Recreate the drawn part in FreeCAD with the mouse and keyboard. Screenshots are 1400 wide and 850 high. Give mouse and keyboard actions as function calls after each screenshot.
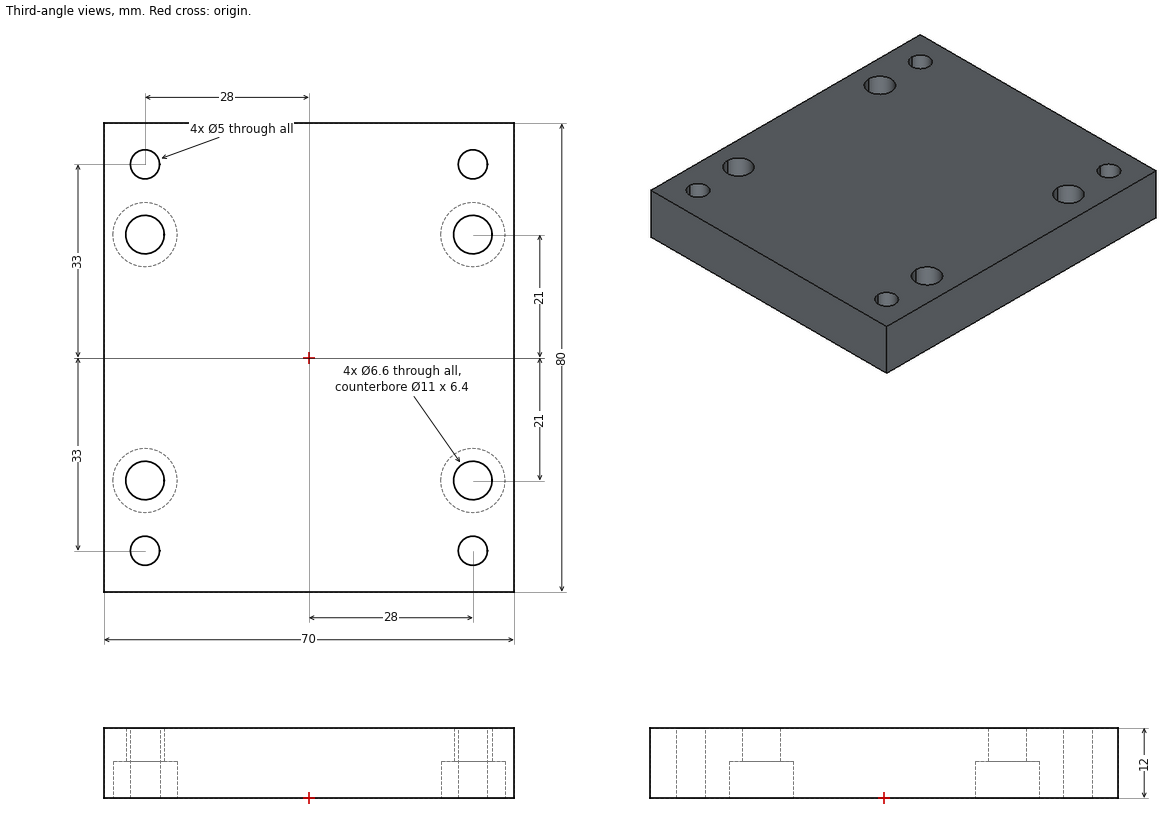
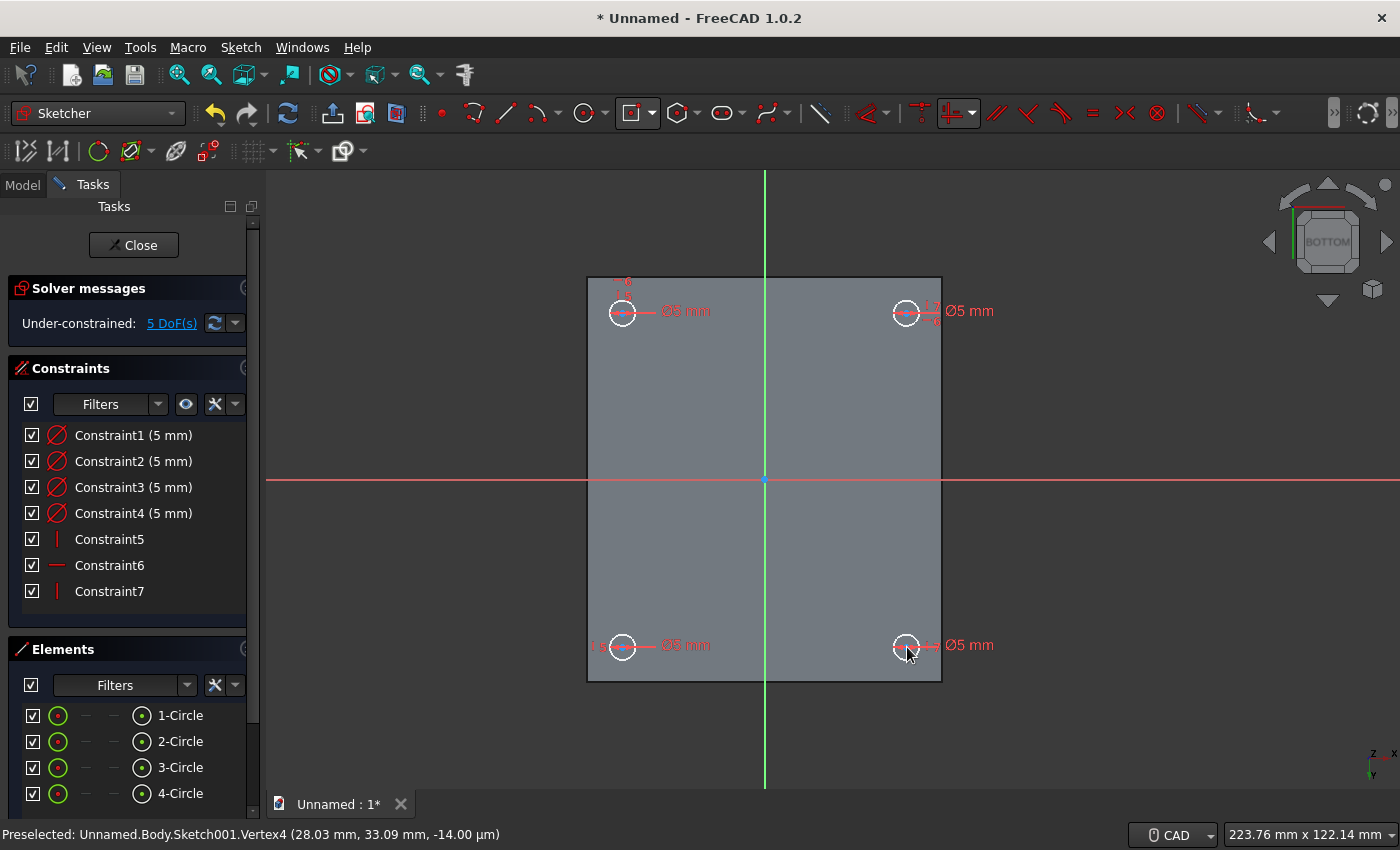
click(623, 647)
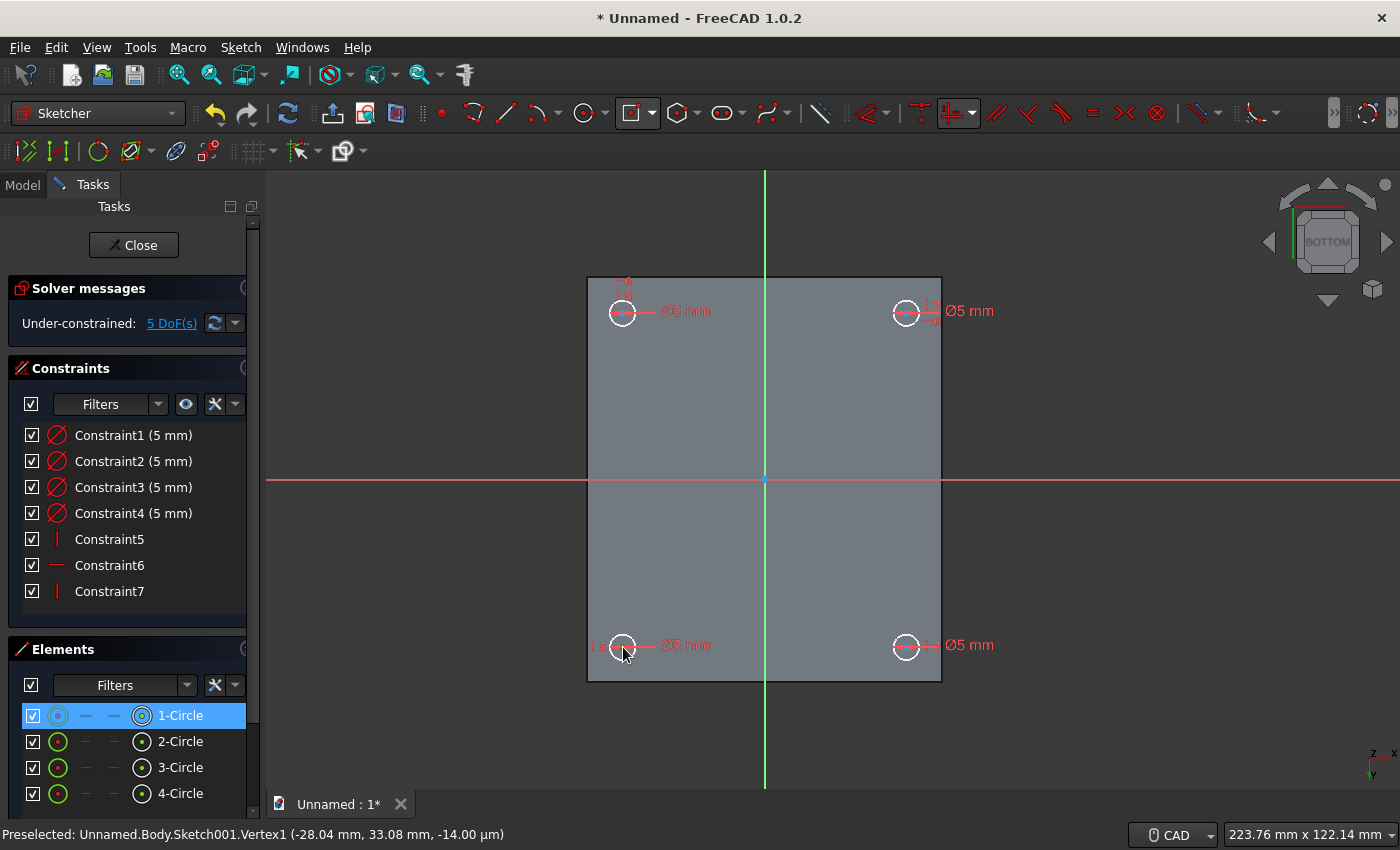
click(906, 647)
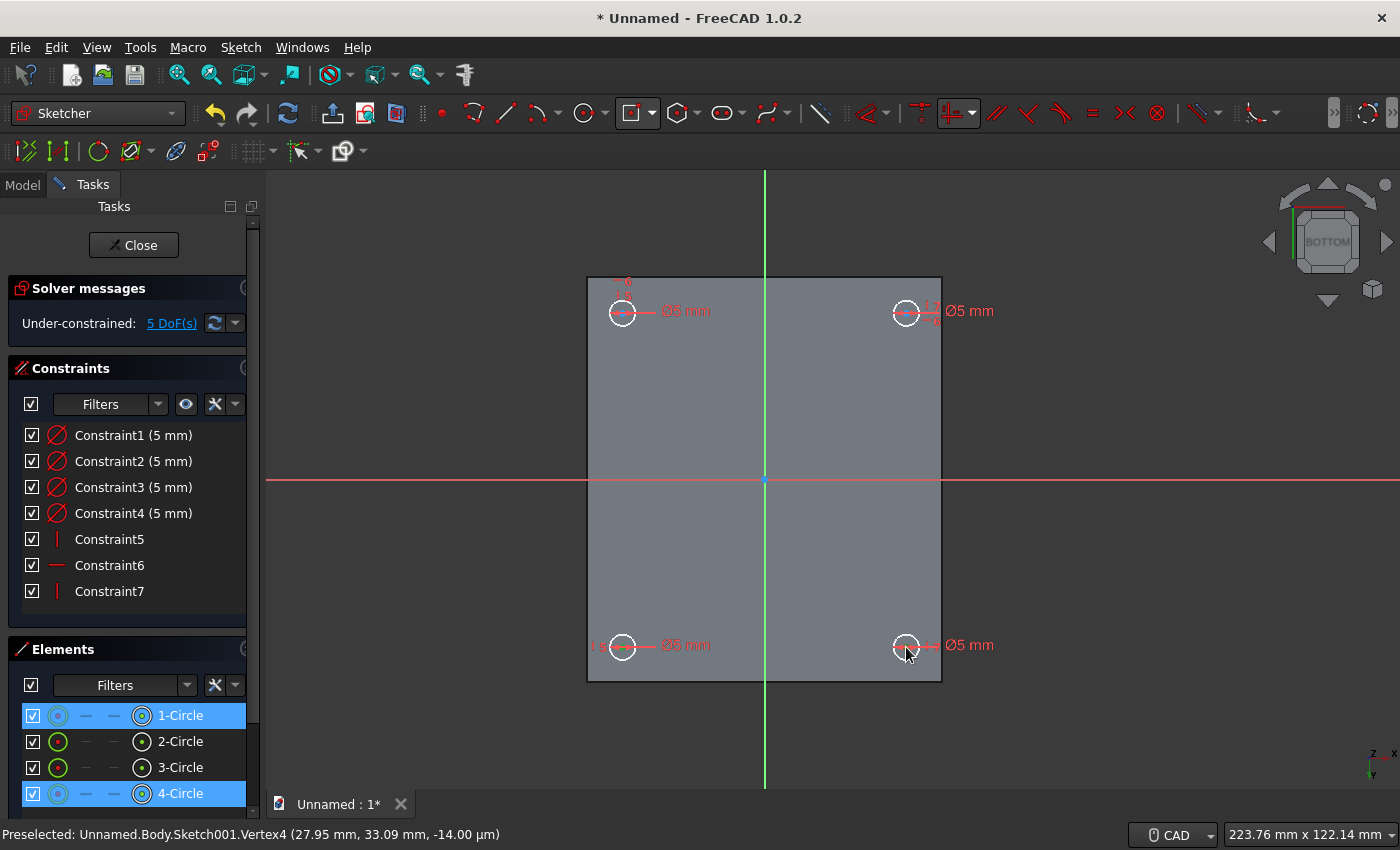
click(974, 114)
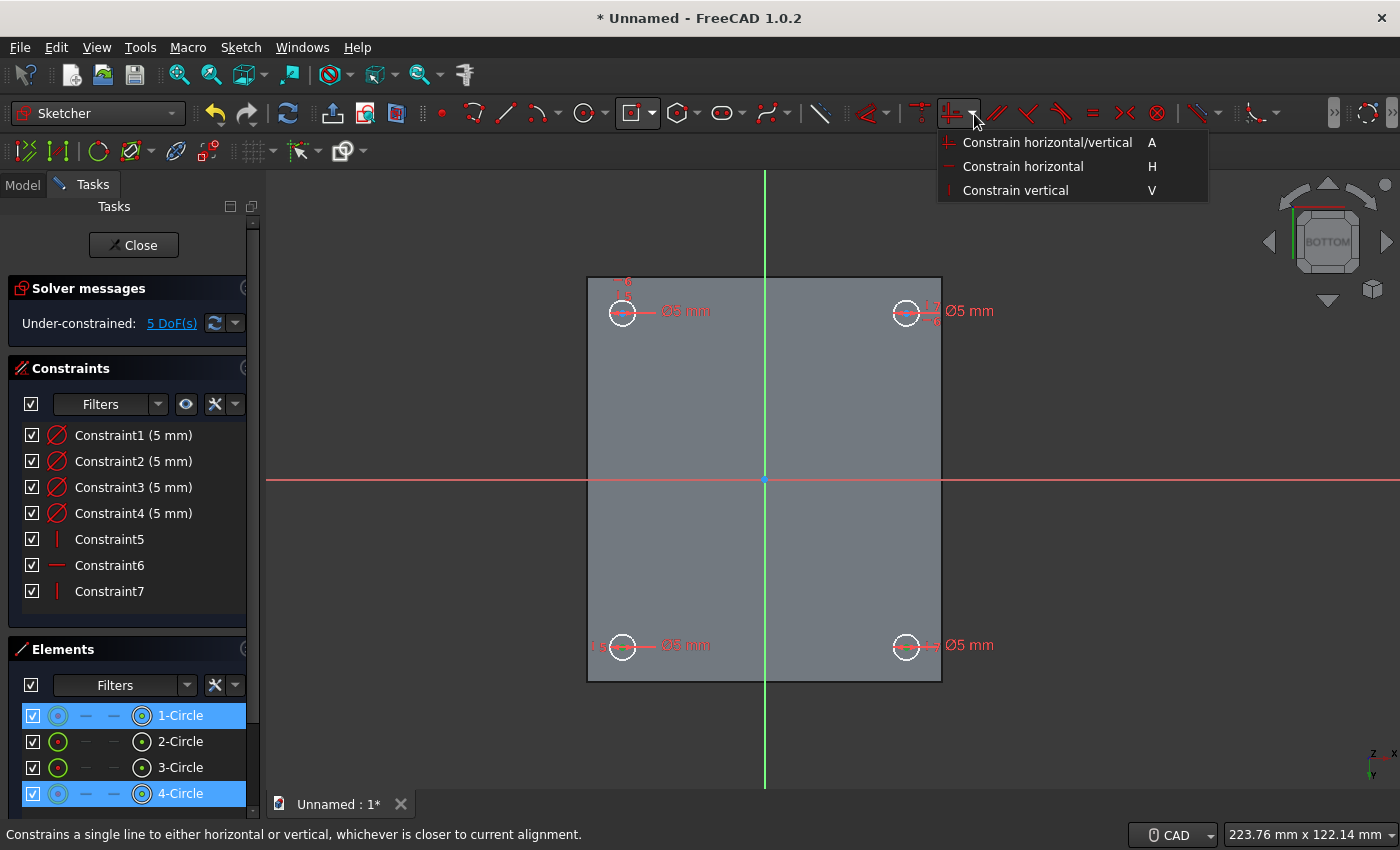
click(1073, 166)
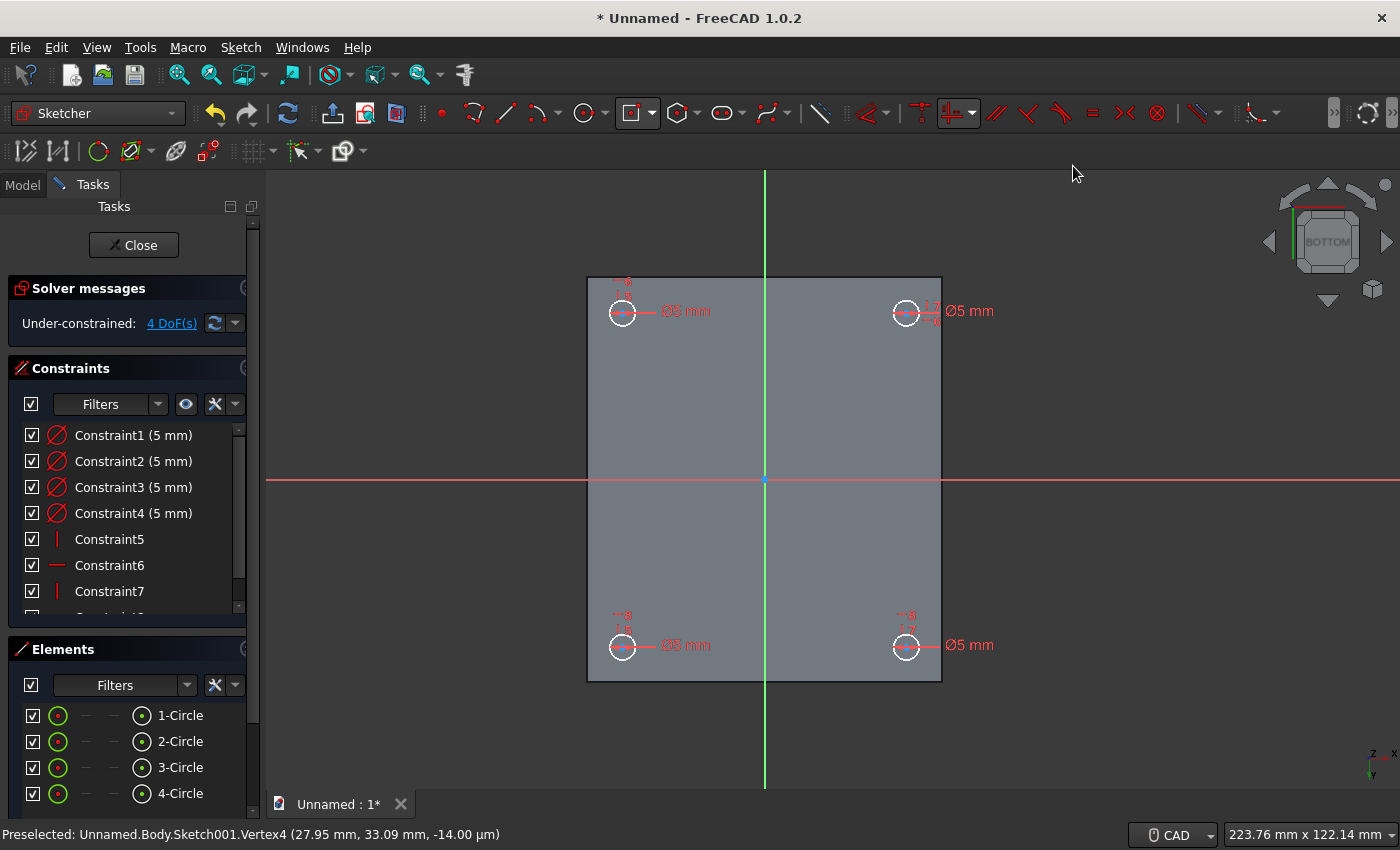
click(623, 647)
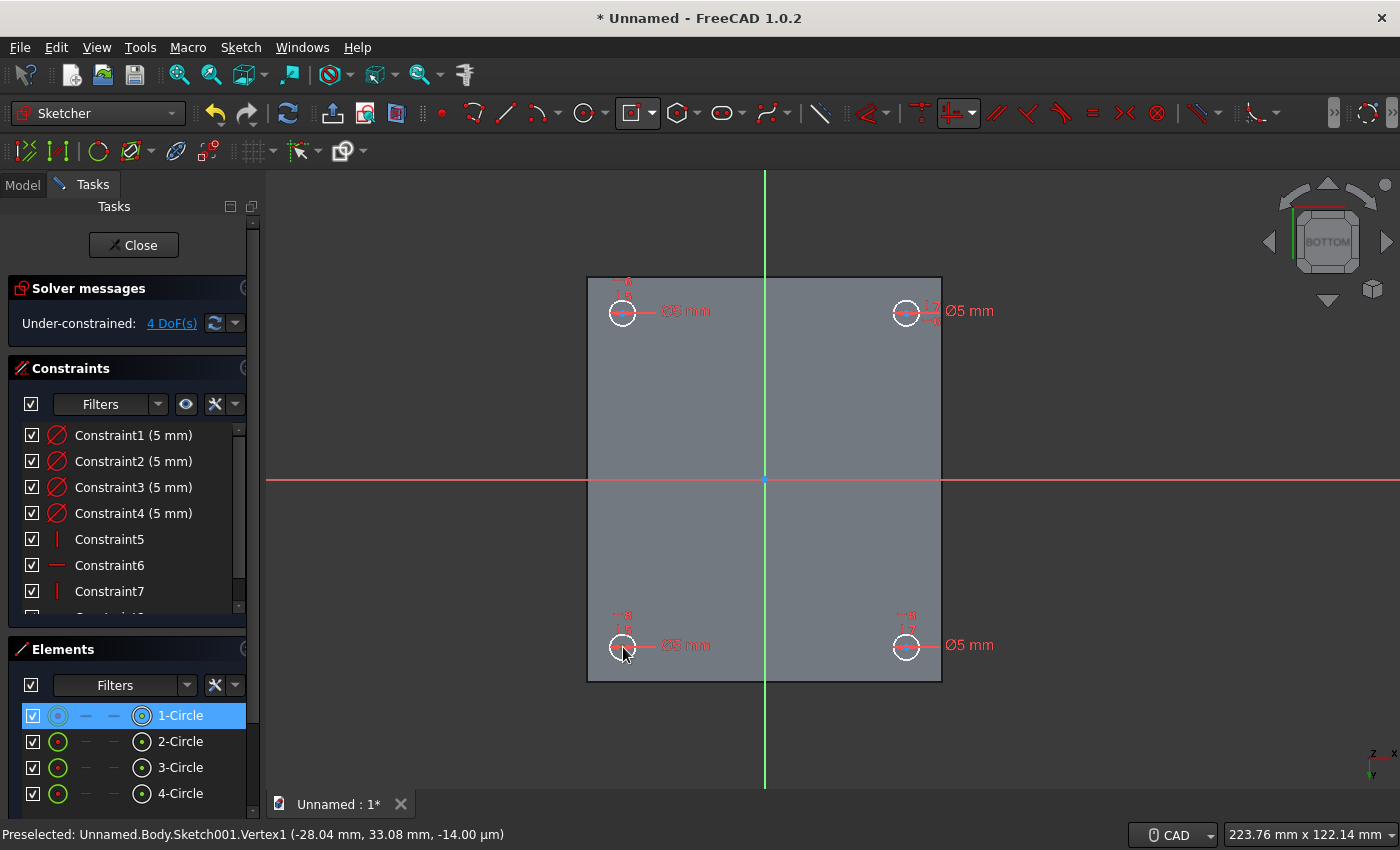
click(888, 114)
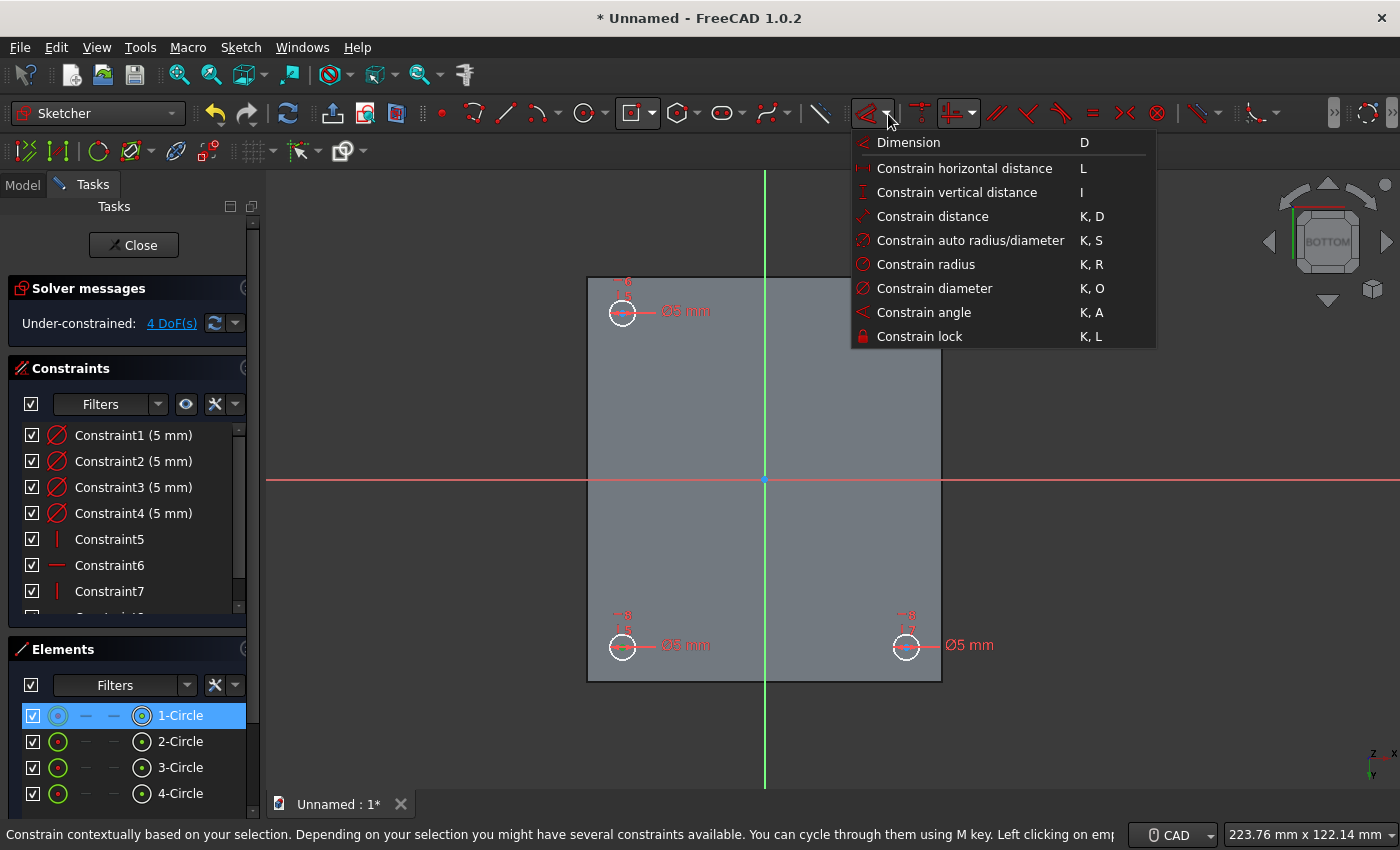
click(1004, 168)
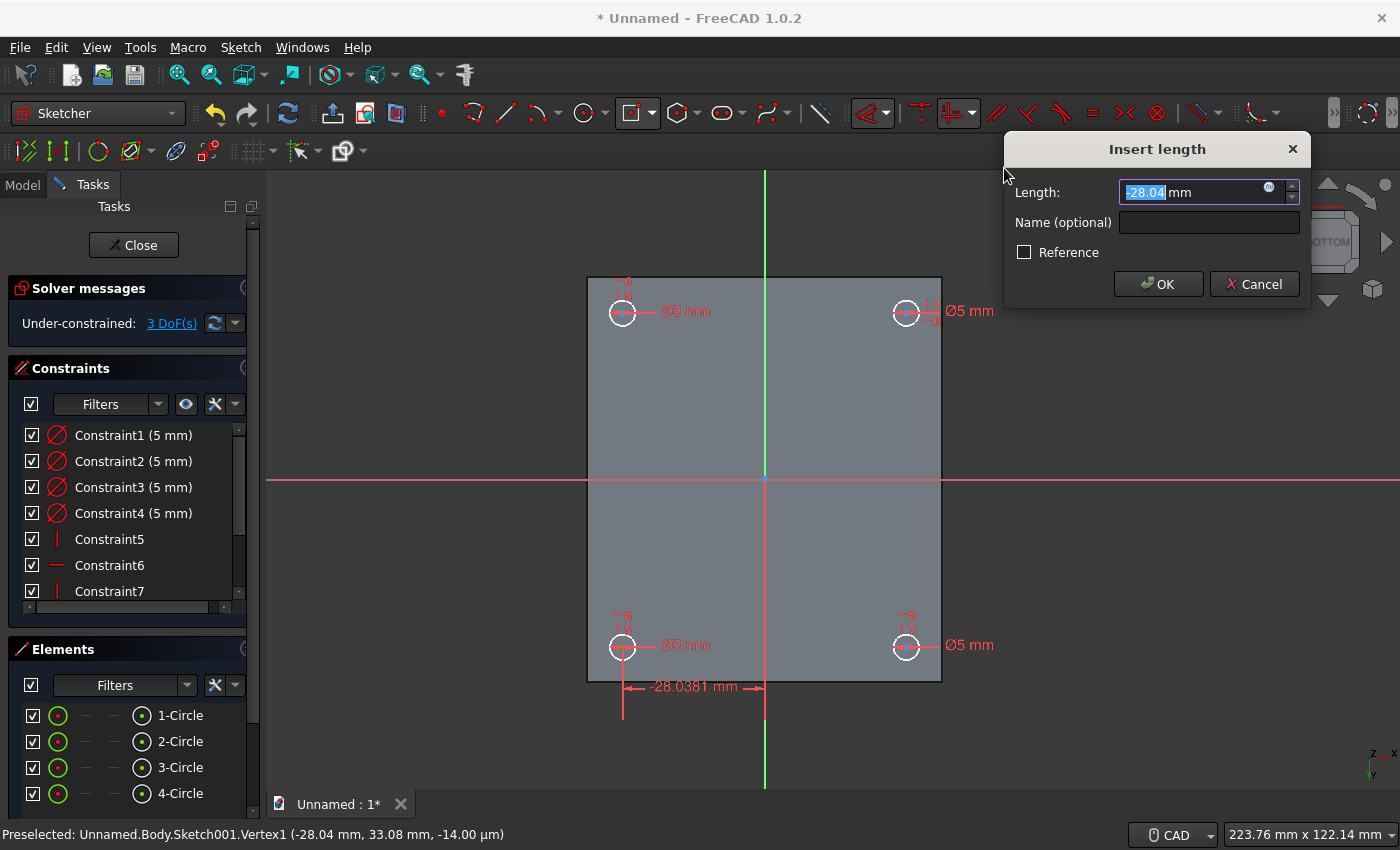
text(-28)
key(Return)